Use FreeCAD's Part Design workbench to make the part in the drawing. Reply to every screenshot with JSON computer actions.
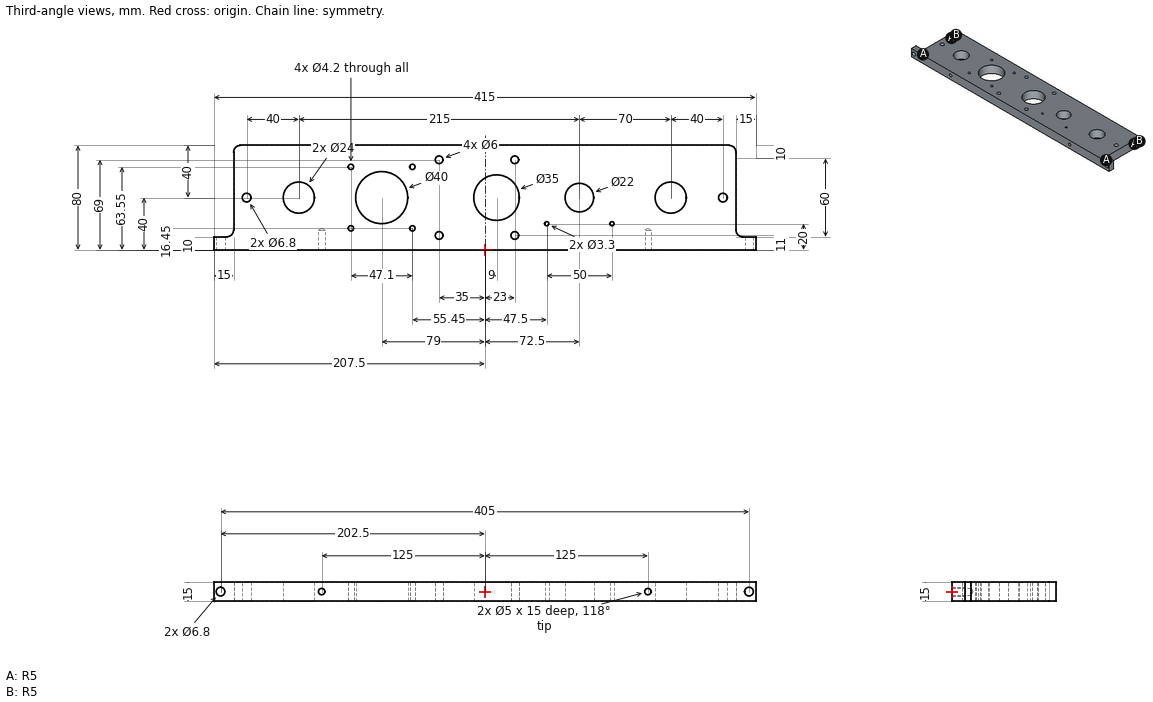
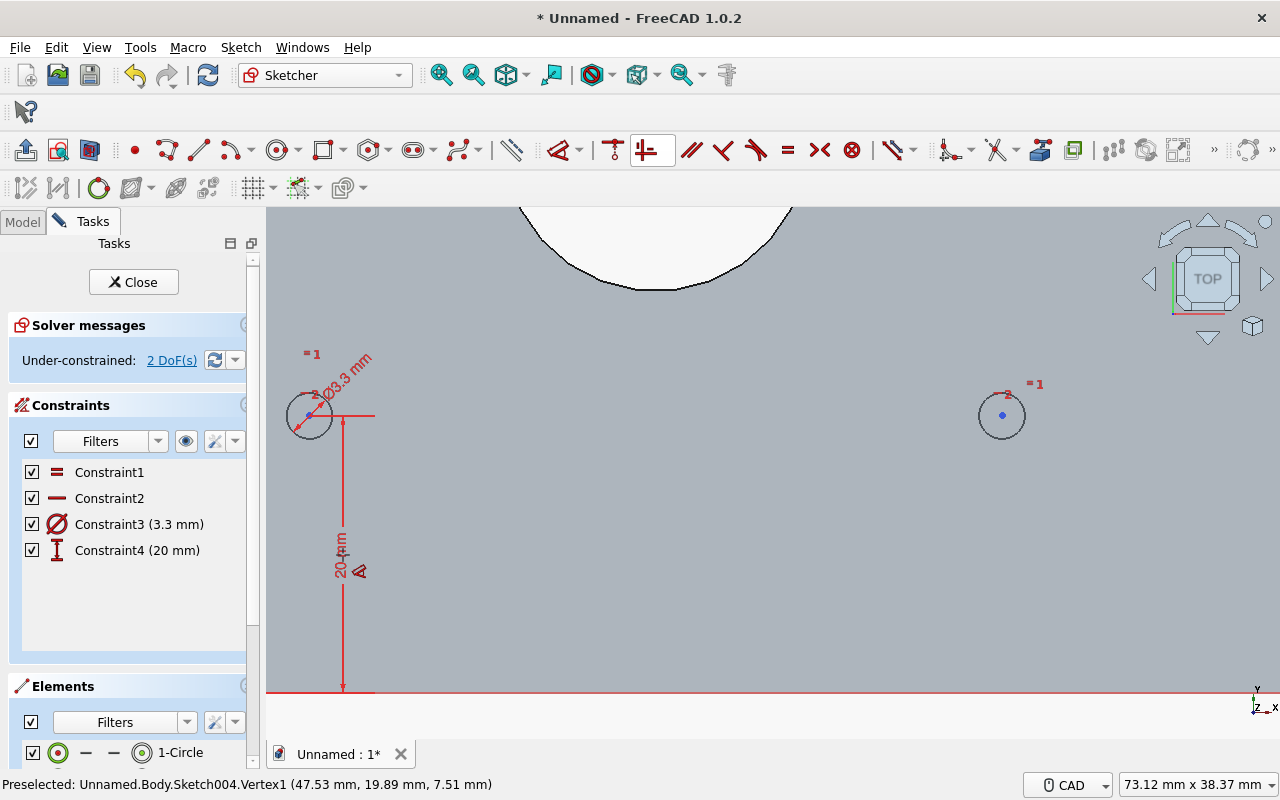
{"action": "left_click", "coordinate": [309, 416]}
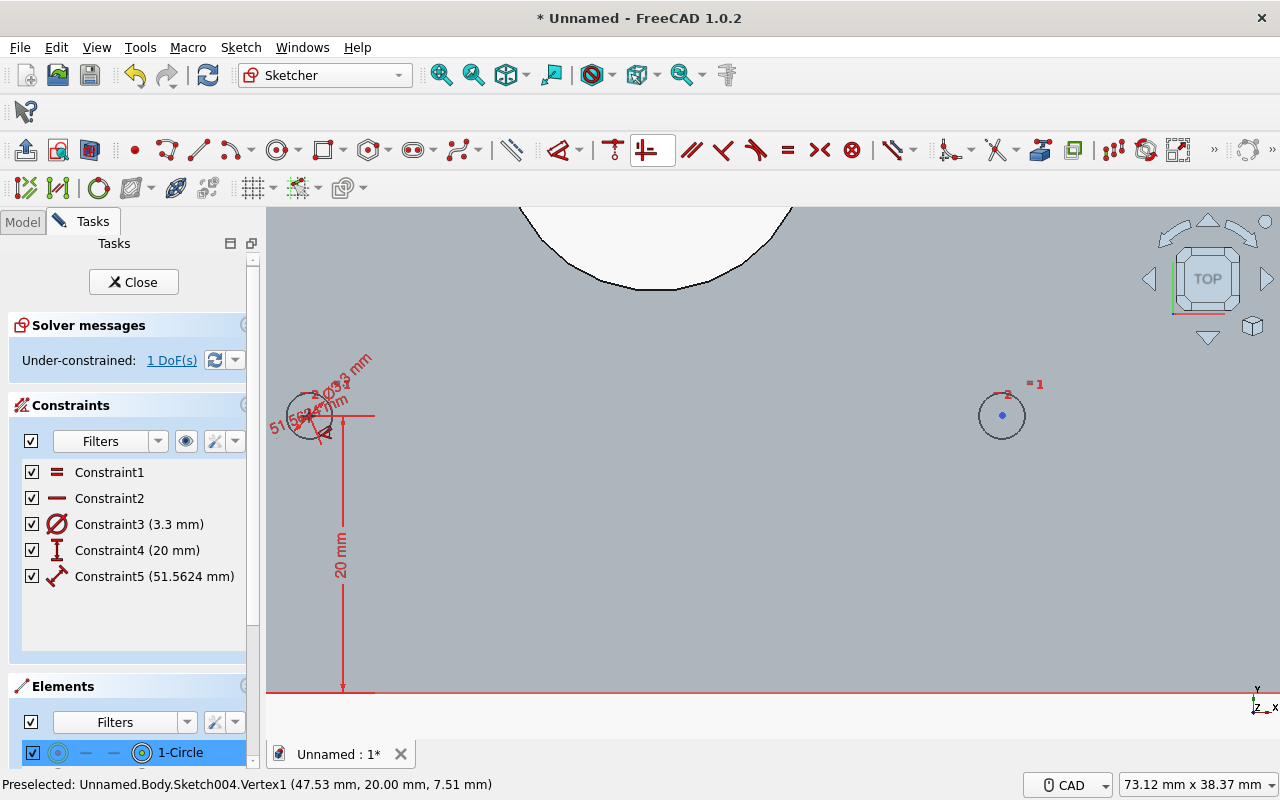
{"action": "left_click", "coordinate": [1002, 416]}
{"action": "left_click", "coordinate": [656, 382]}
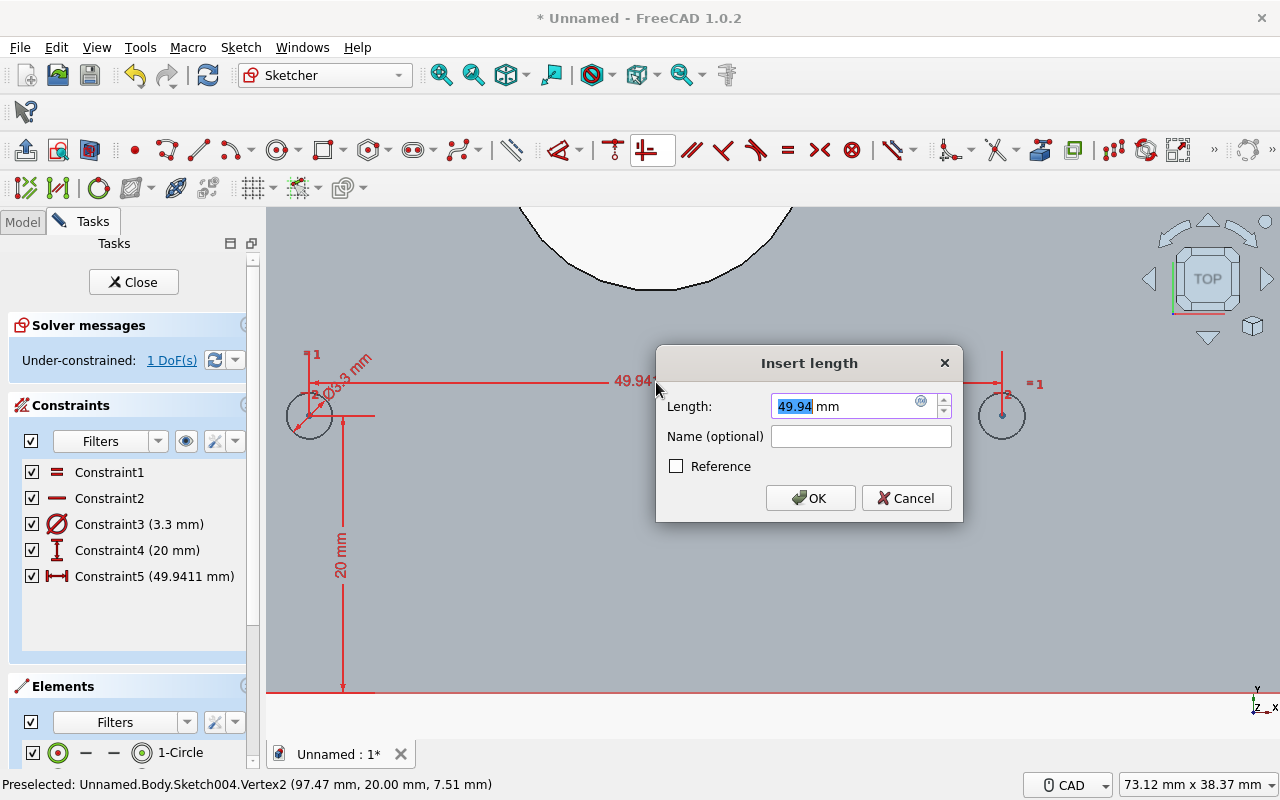
{"action": "type", "text": "50"}
{"action": "key", "text": "Return"}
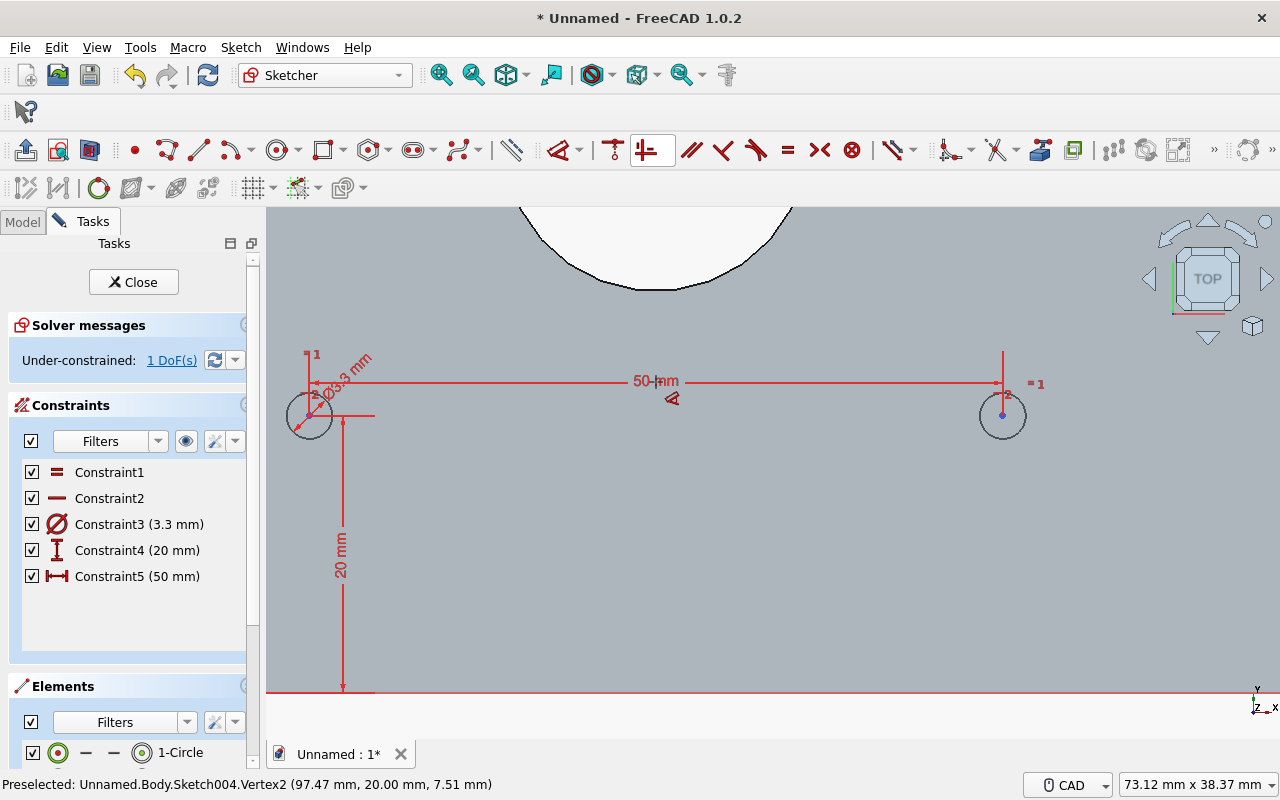
{"action": "left_click", "coordinate": [309, 416]}
{"action": "left_click", "coordinate": [302, 358]}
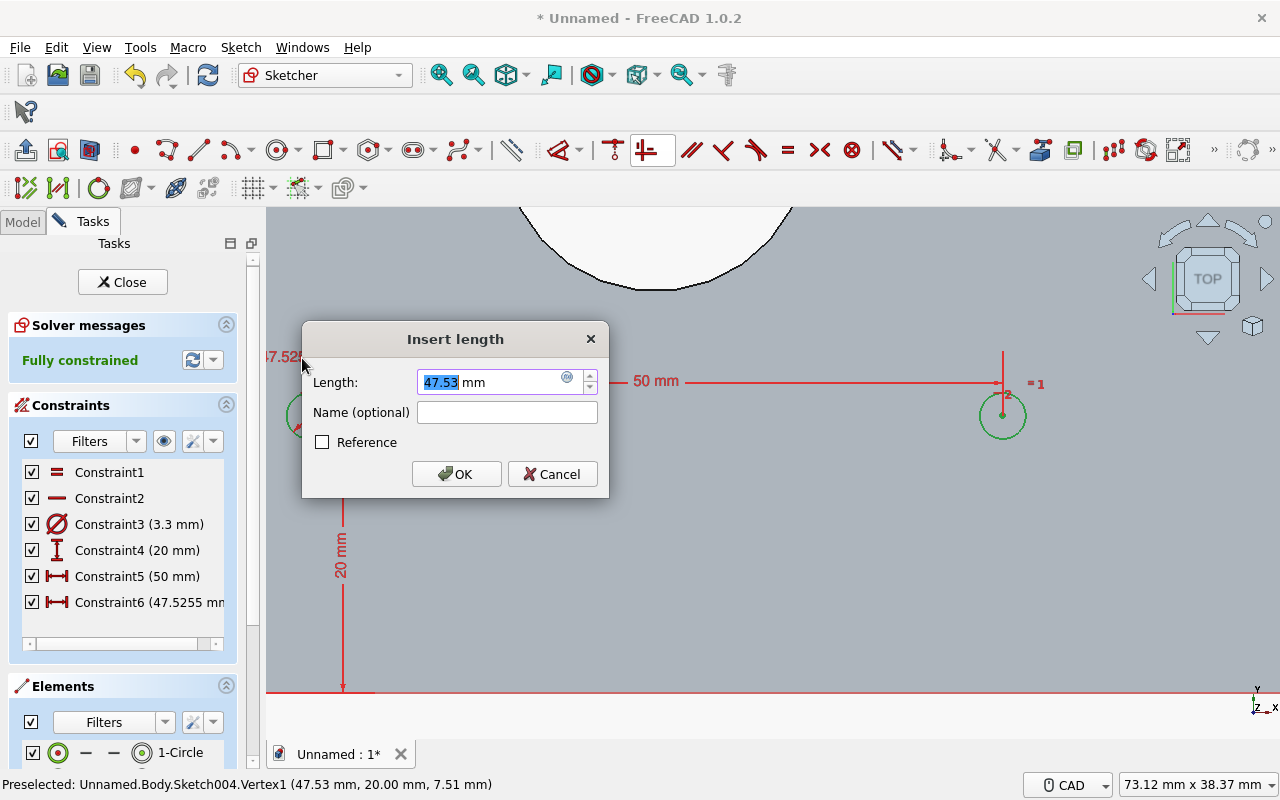
{"action": "type", "text": "47.5"}
{"action": "key", "text": "Return"}
{"action": "key", "text": "Escape"}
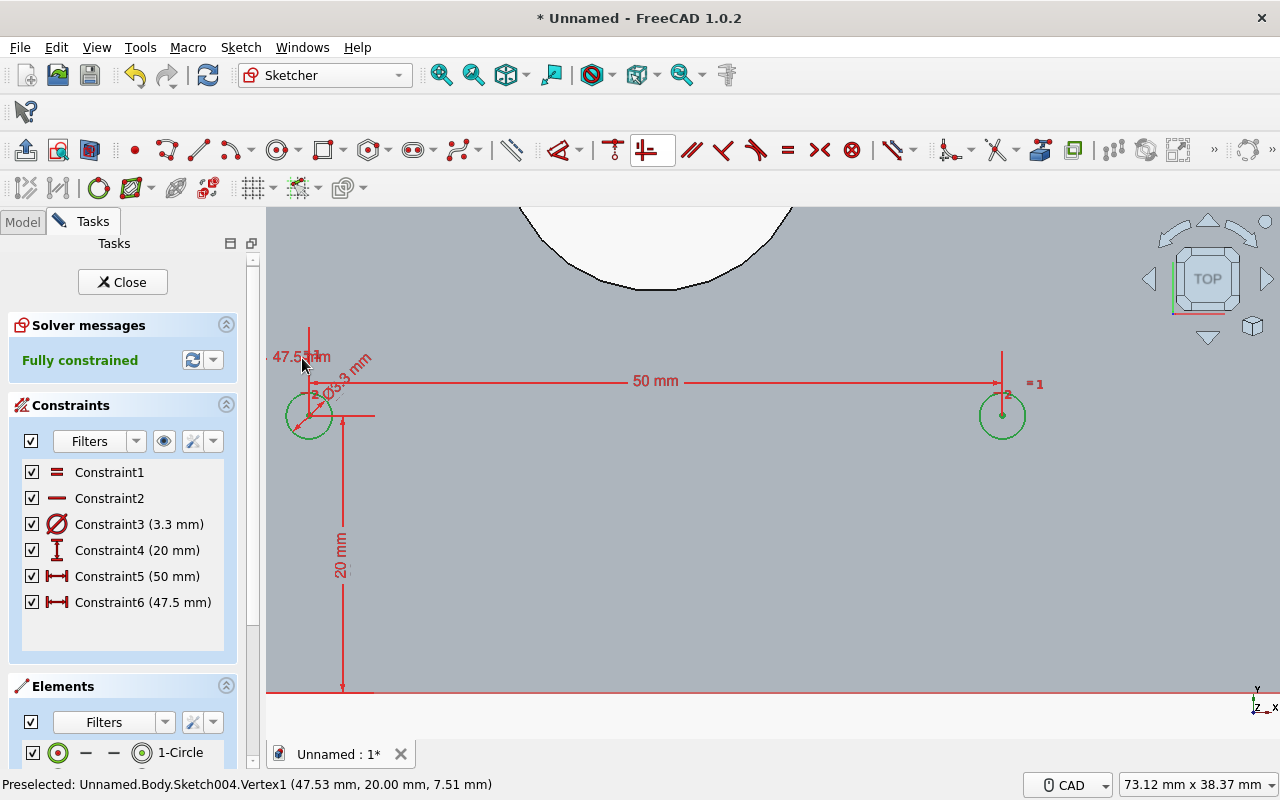
{"action": "left_click", "coordinate": [123, 282]}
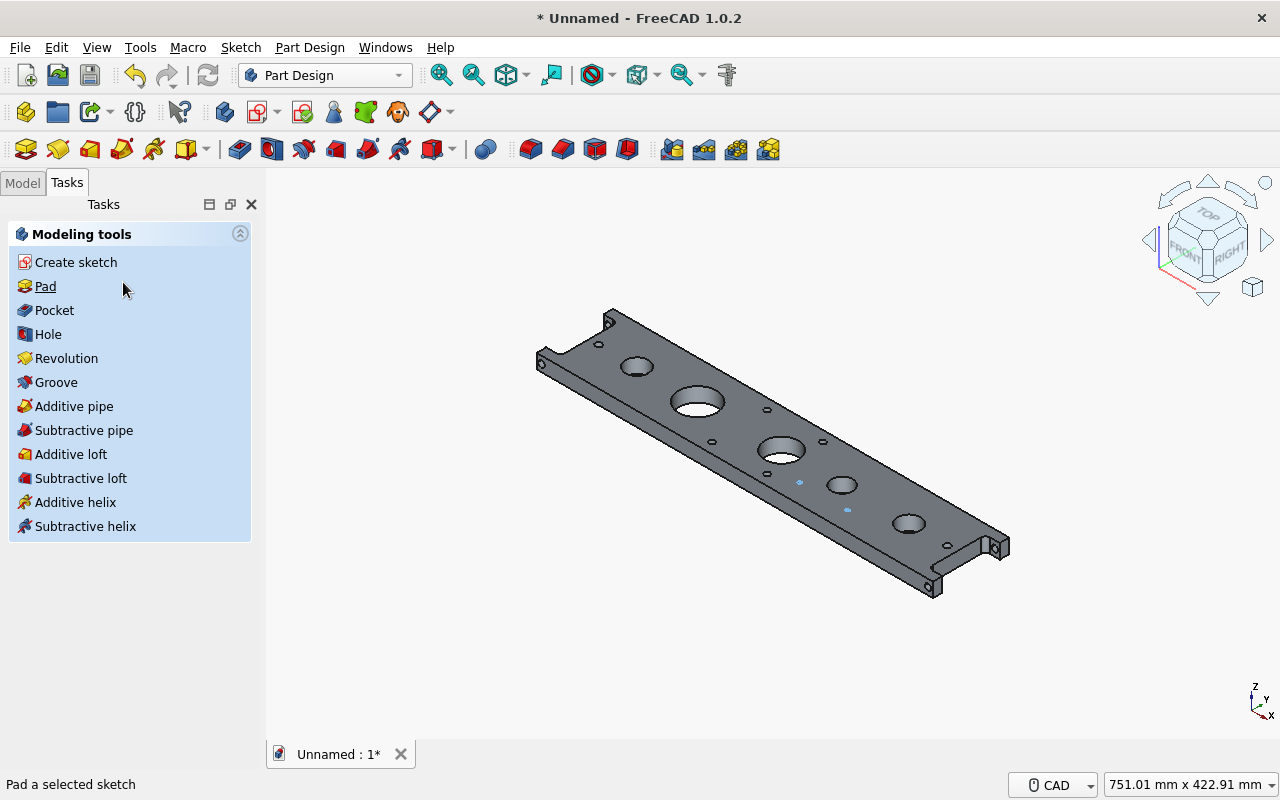
{"action": "left_click", "coordinate": [240, 150]}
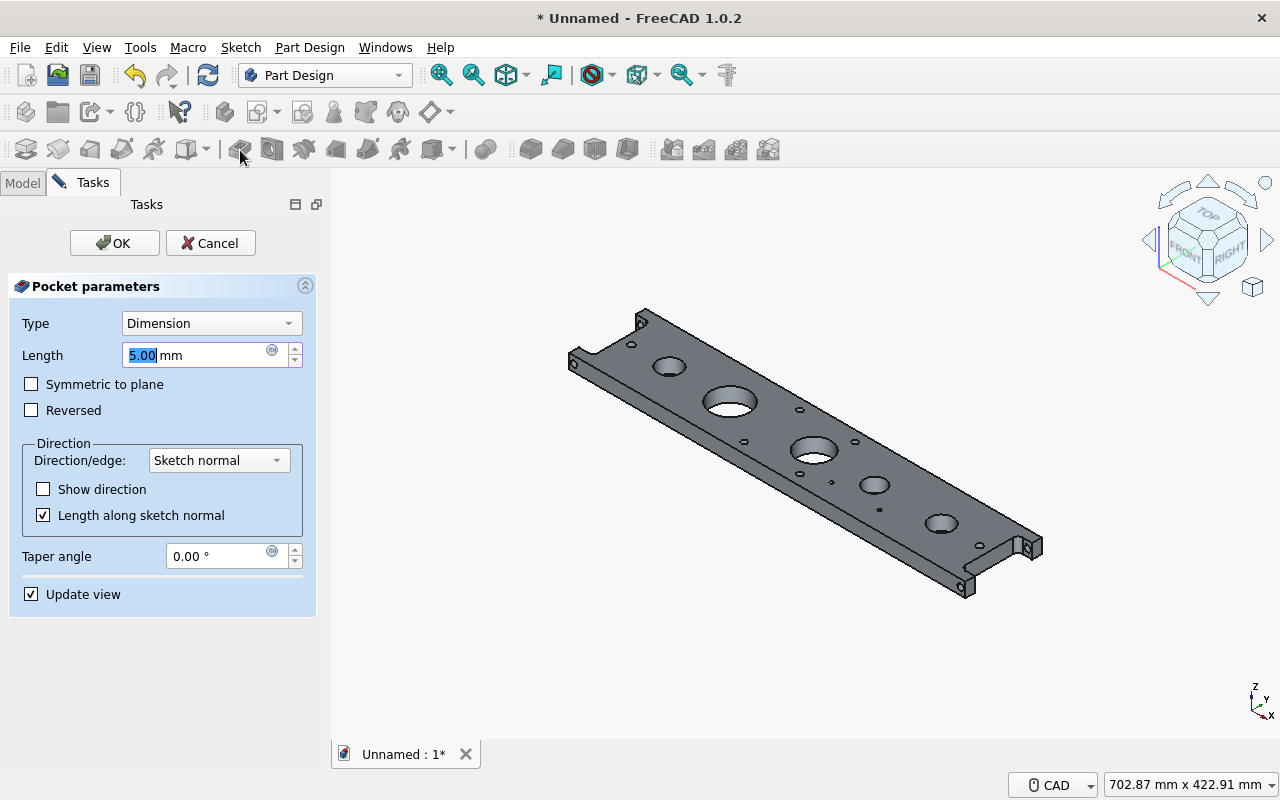
{"action": "left_click", "coordinate": [212, 324]}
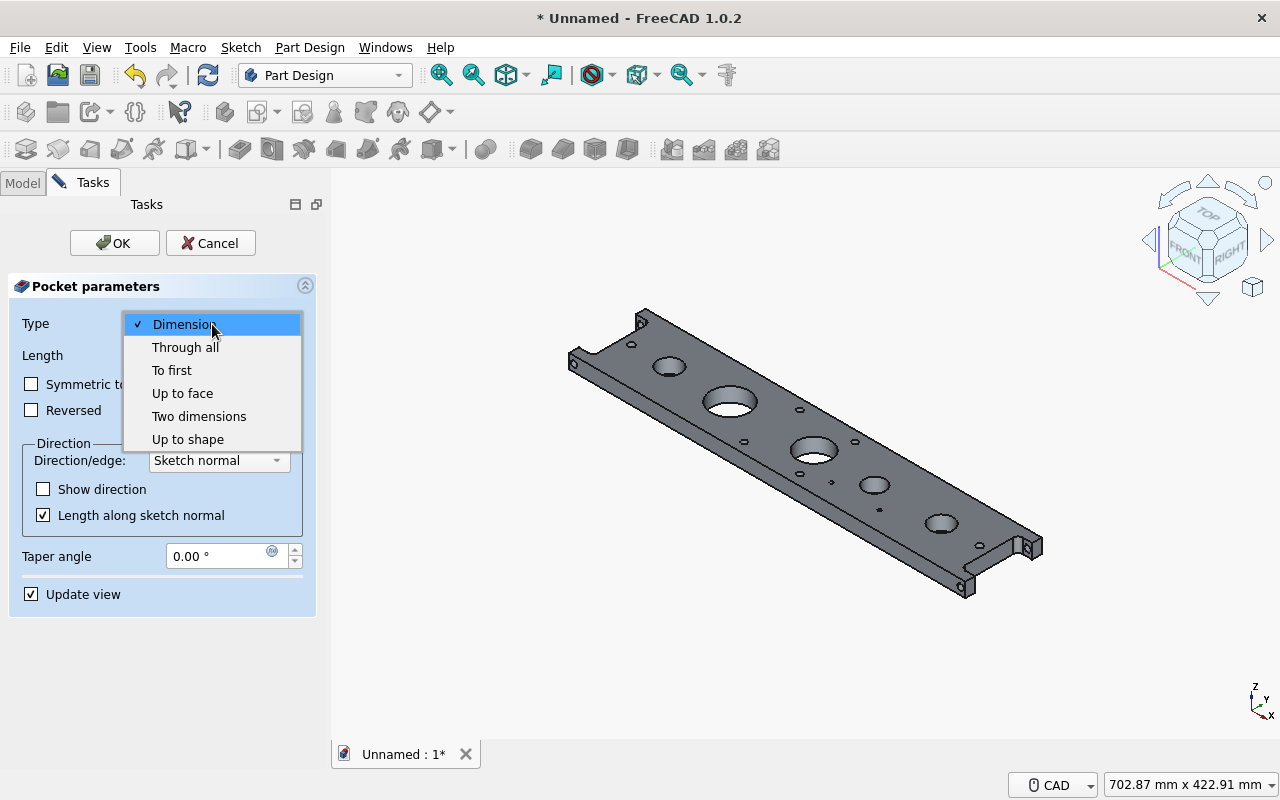
{"action": "left_click", "coordinate": [212, 348]}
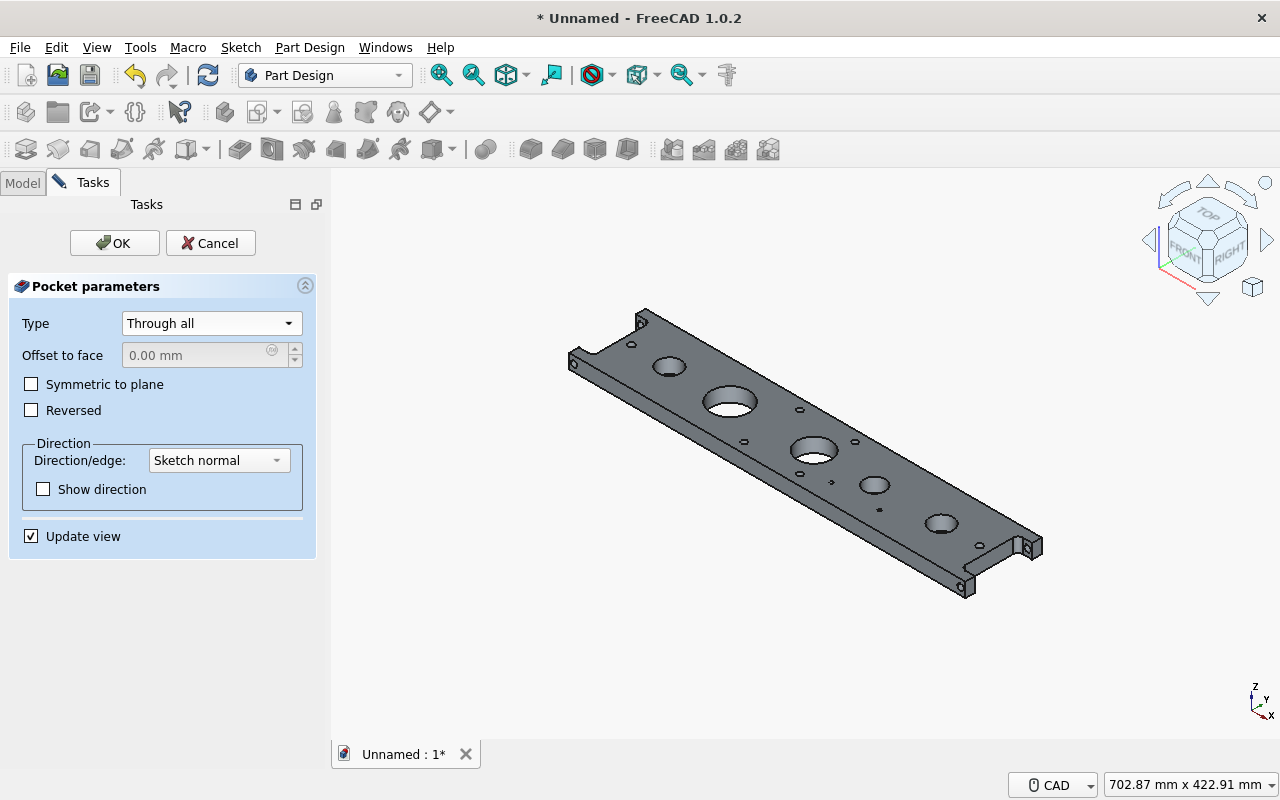
{"action": "left_click", "coordinate": [115, 243]}